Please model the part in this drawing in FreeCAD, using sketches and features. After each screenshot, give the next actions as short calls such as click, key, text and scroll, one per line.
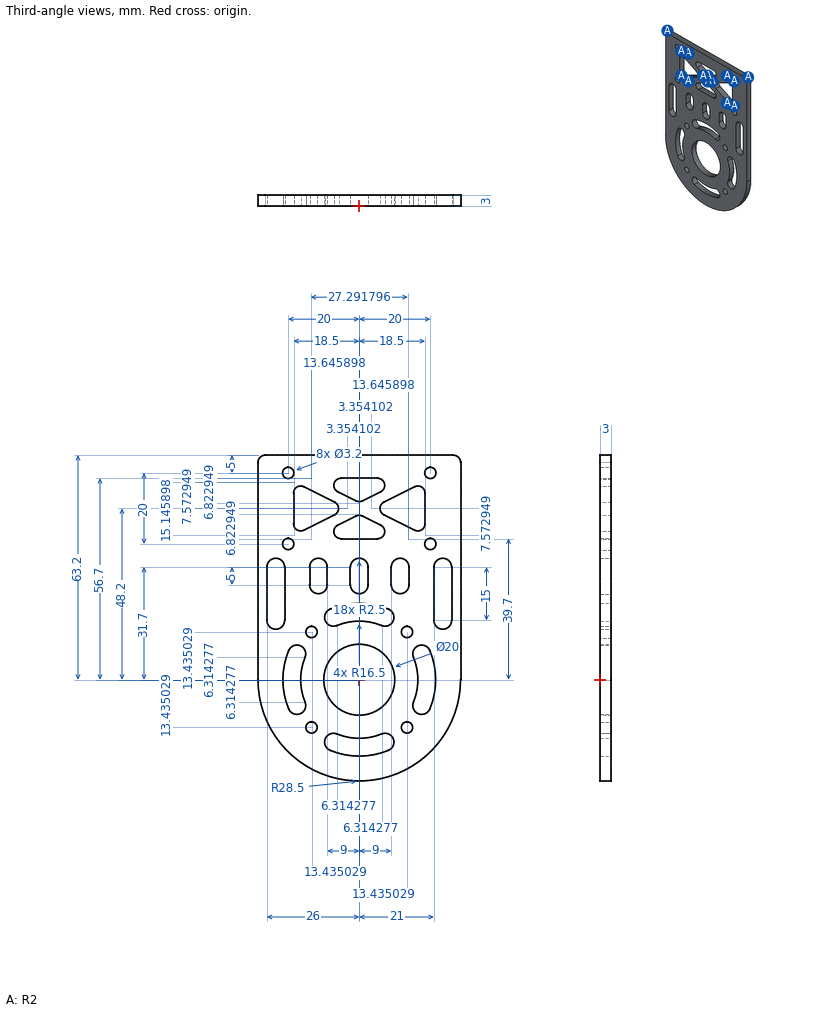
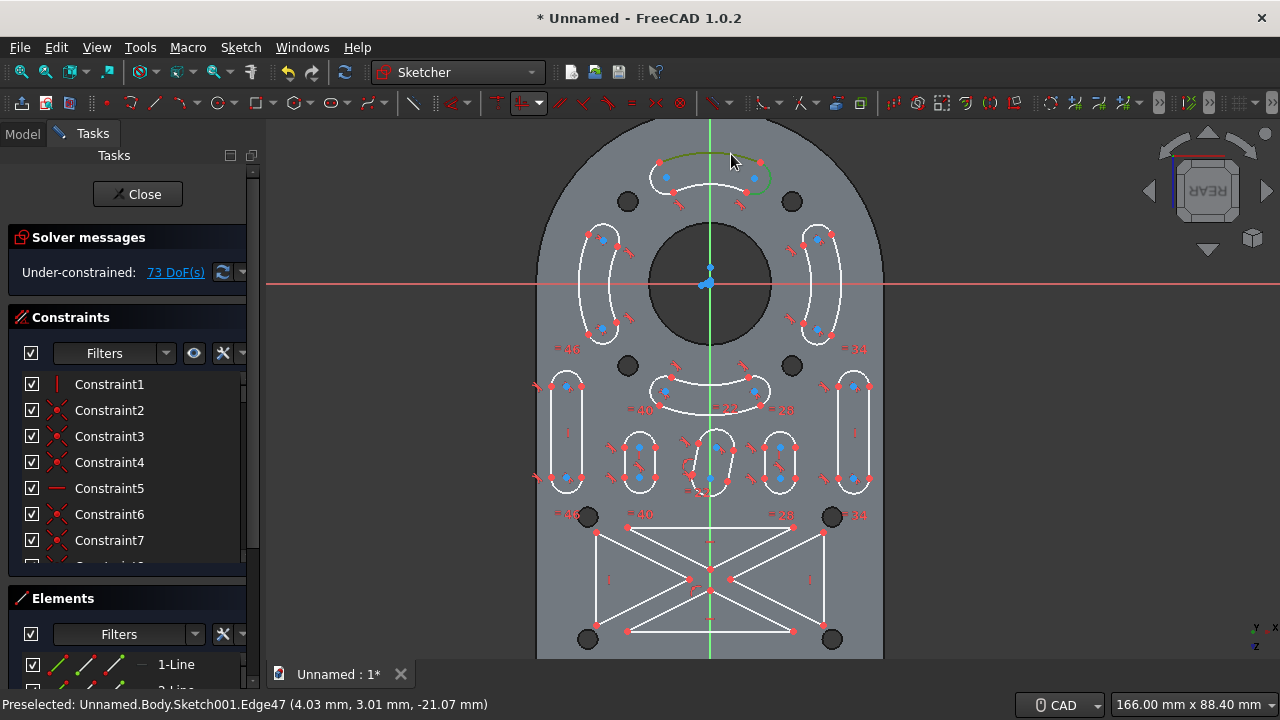
key(t)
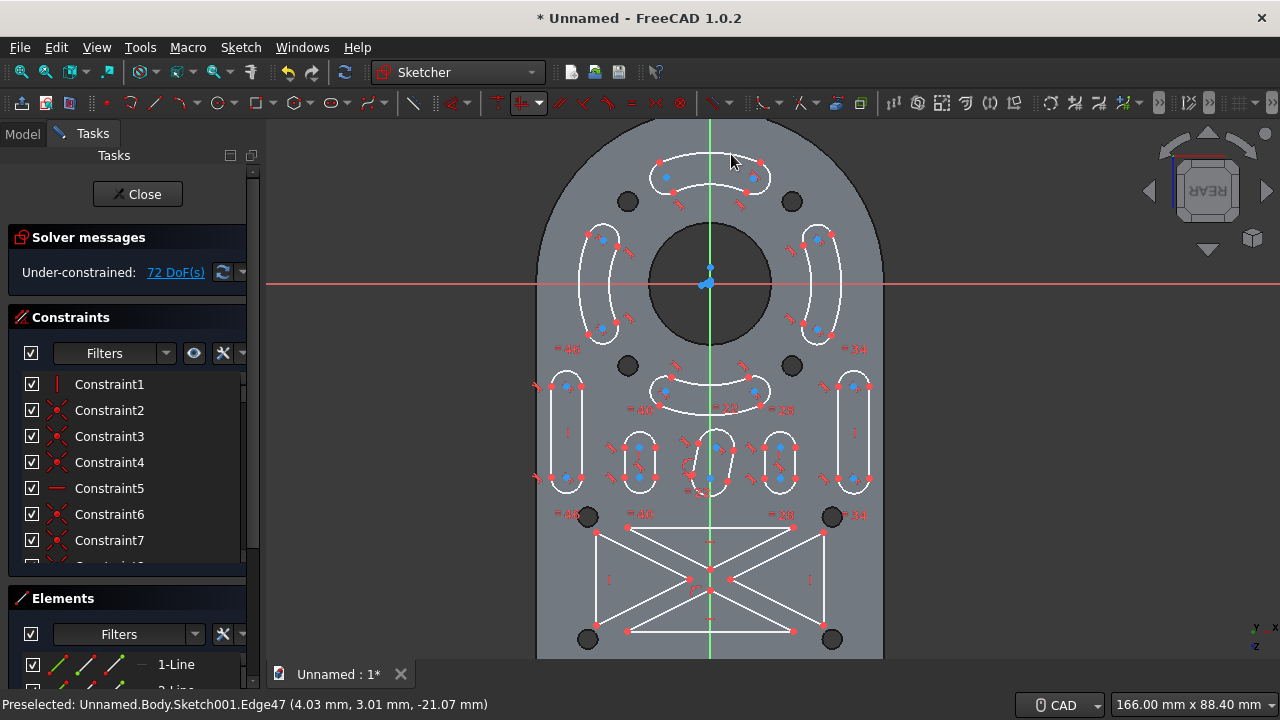
click(731, 154)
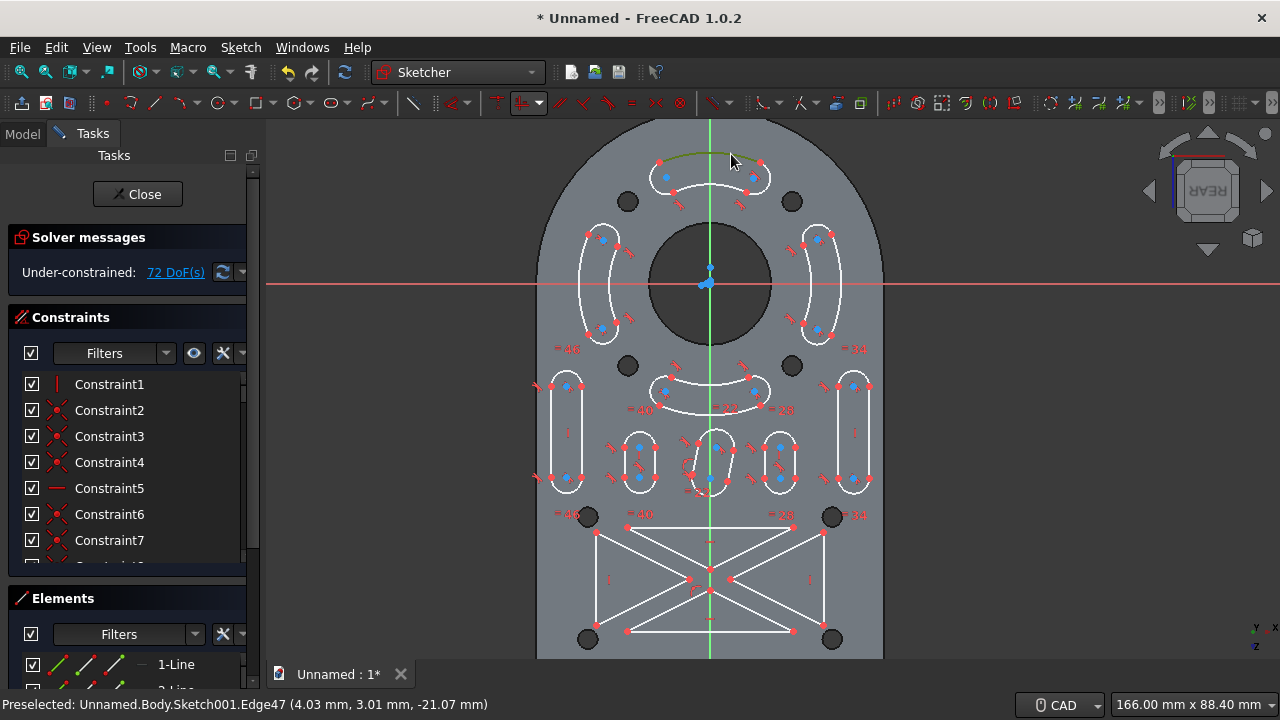
click(651, 175)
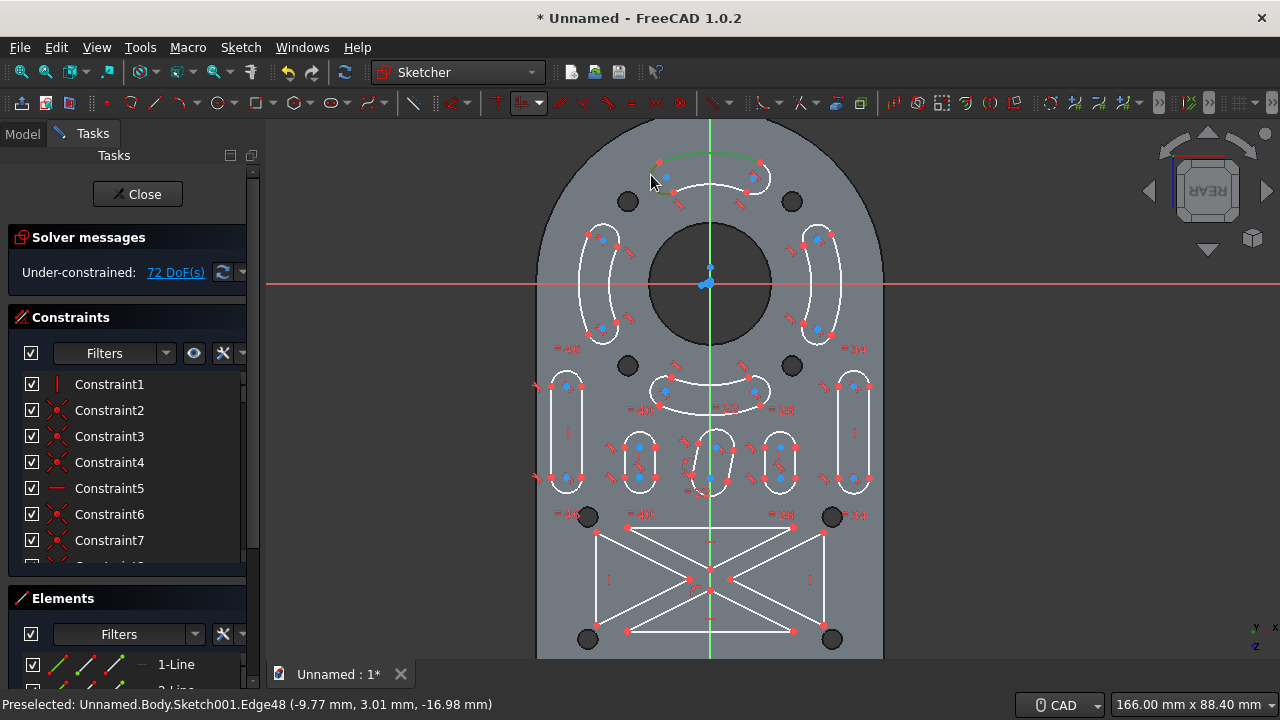
key(t)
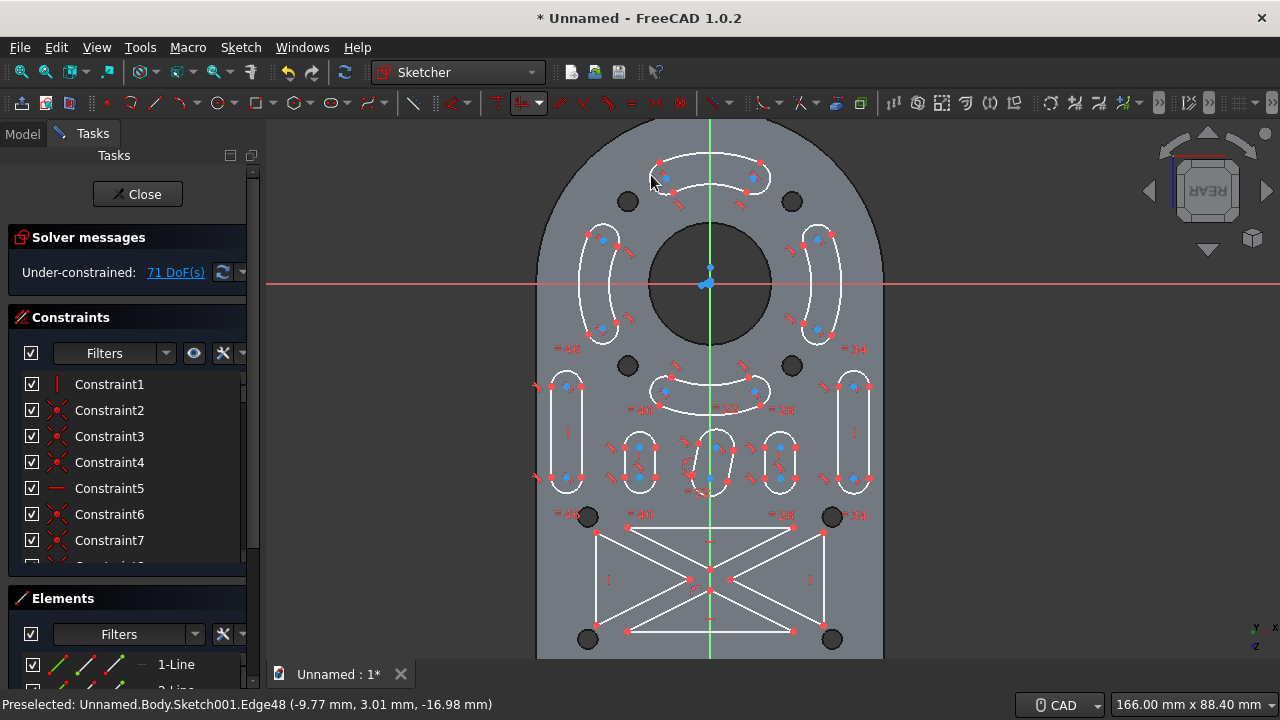
scroll(694, 465, up, 2)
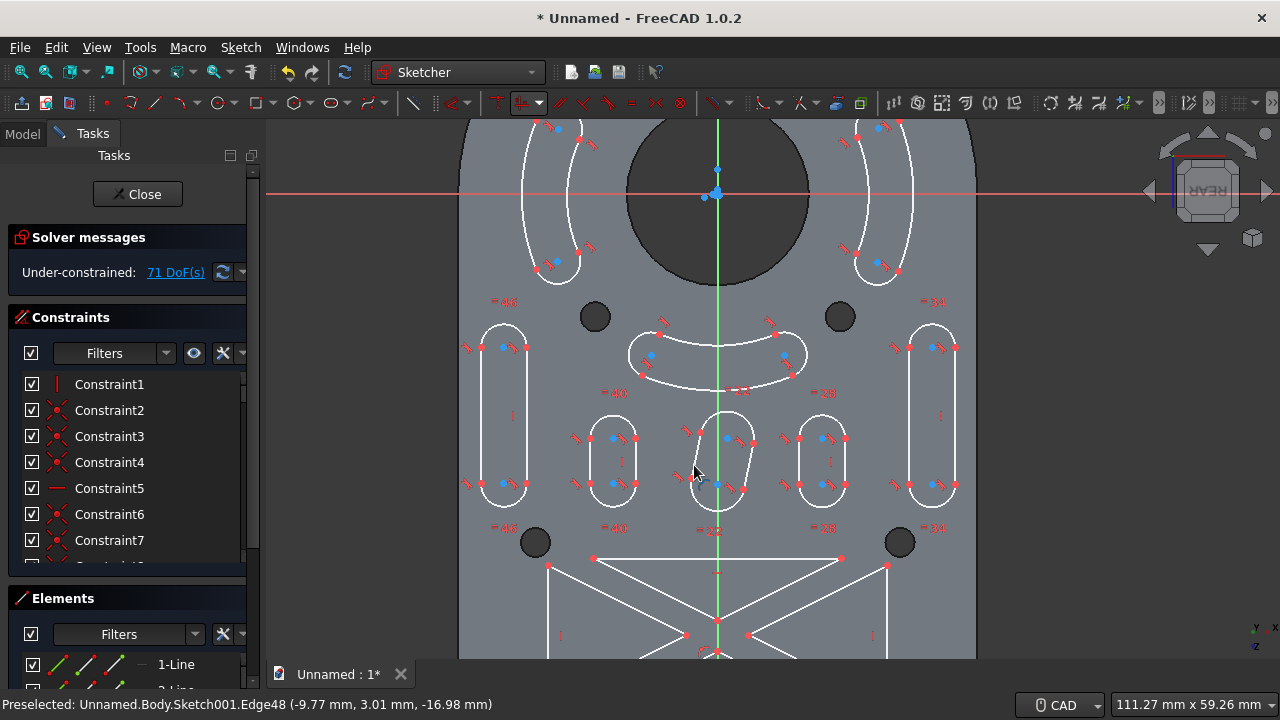
click(694, 465)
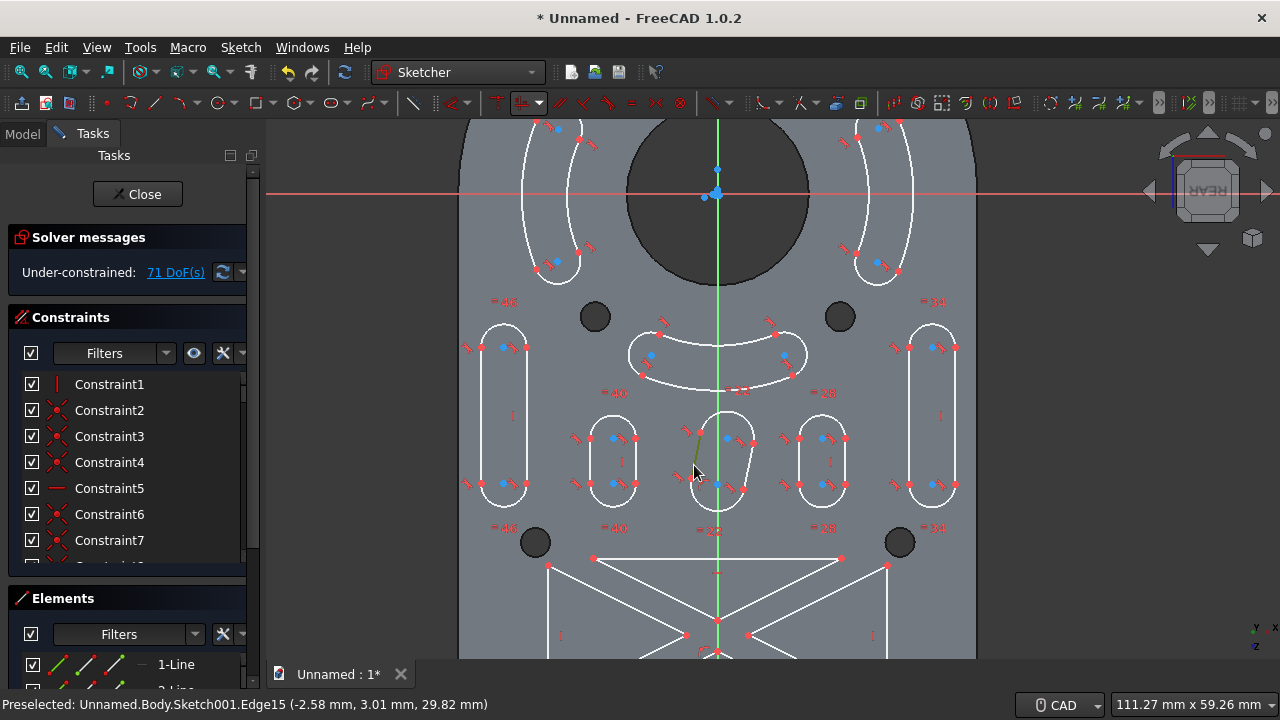
key(v)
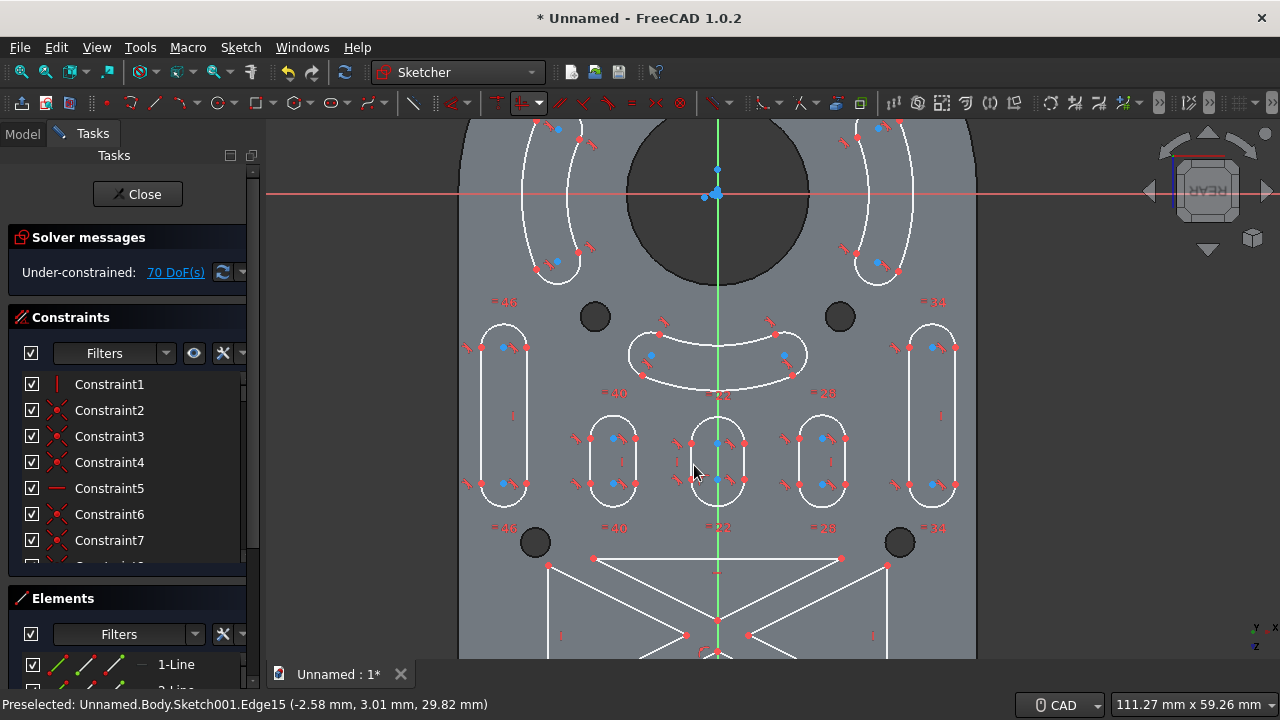
click(694, 344)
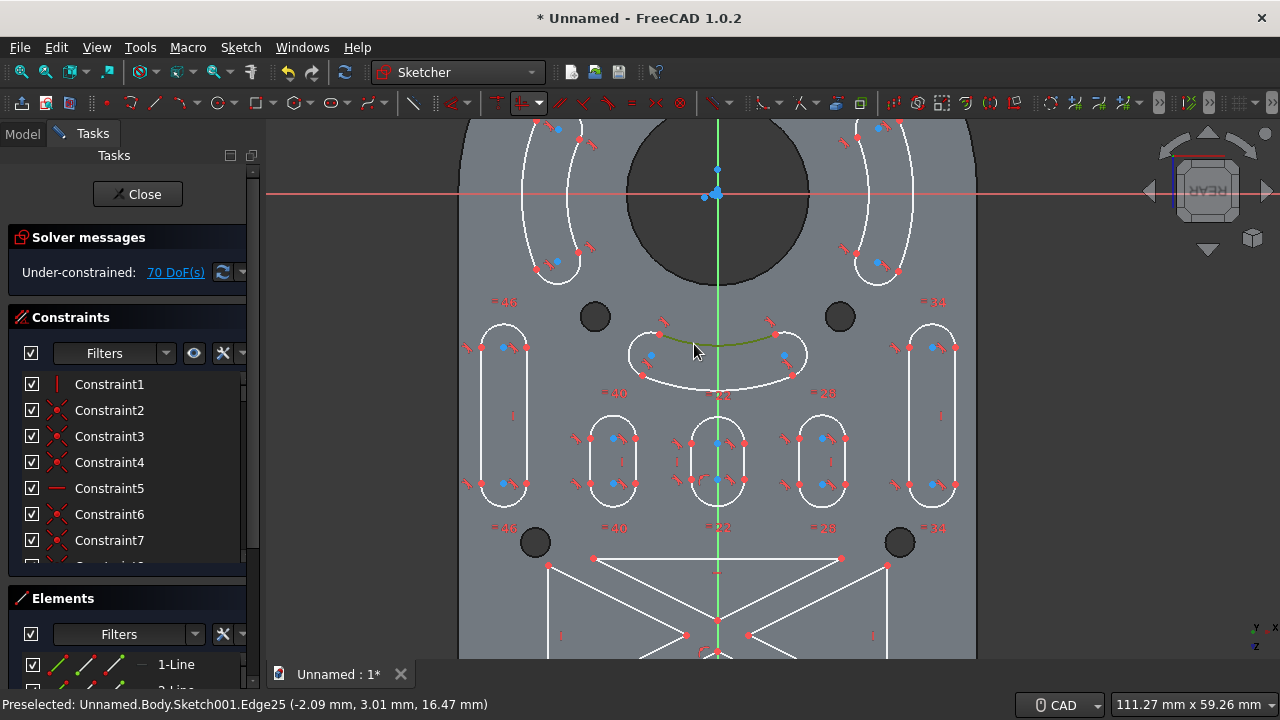
click(687, 388)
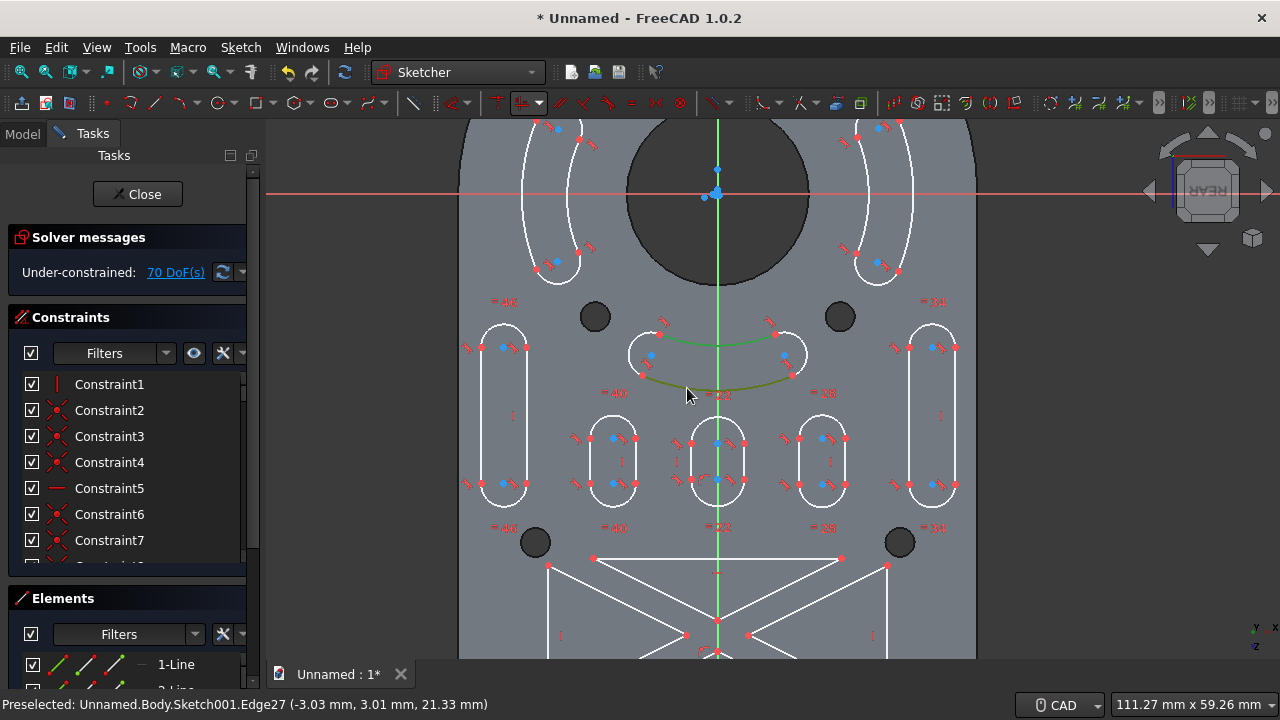
click(498, 104)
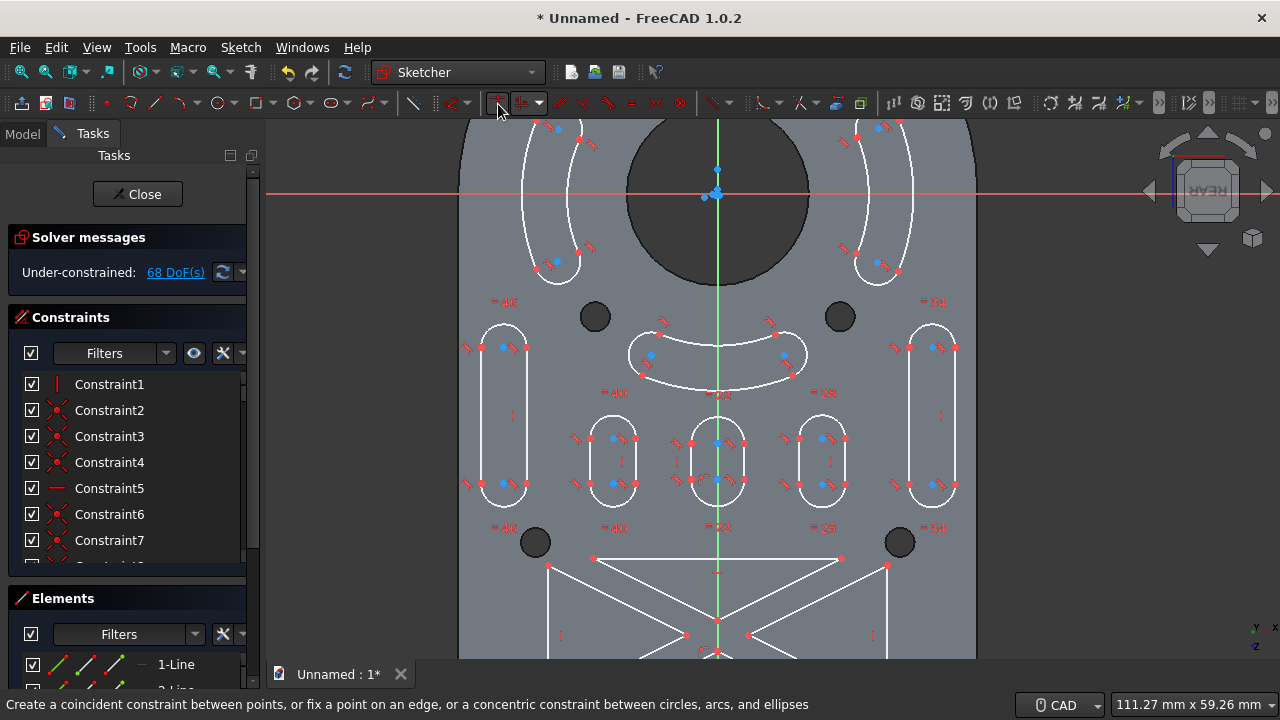
click(694, 344)